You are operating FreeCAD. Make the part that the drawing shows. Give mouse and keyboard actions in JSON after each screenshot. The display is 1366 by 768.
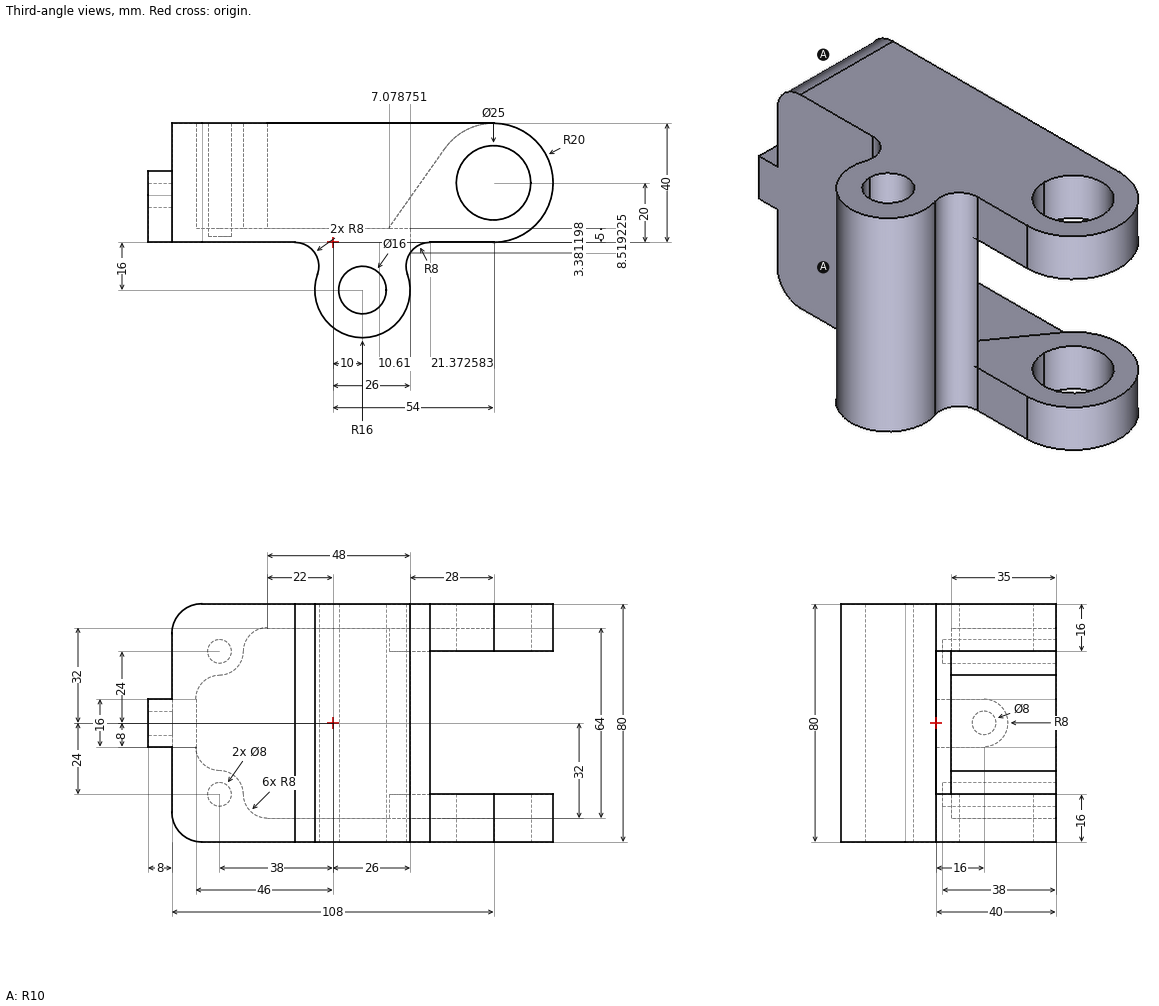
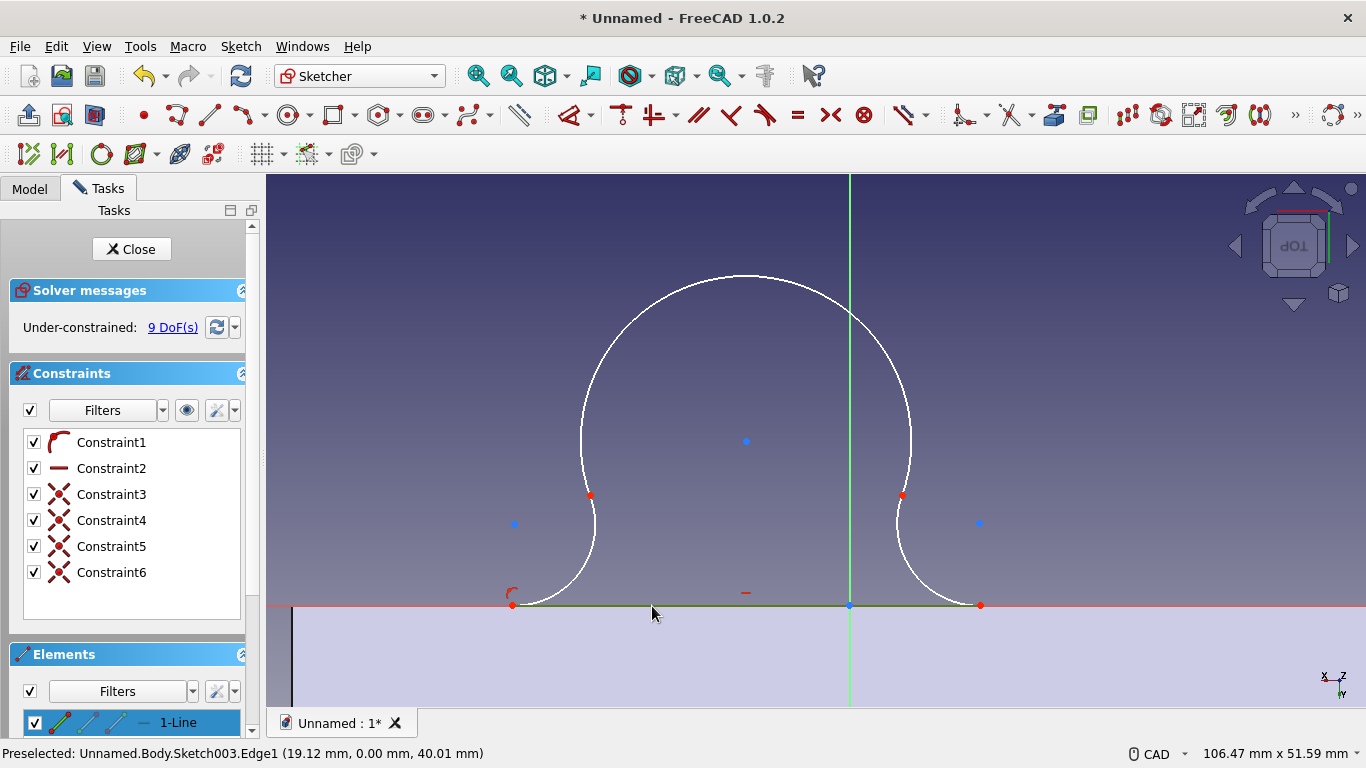
{"action": "left_click", "coordinate": [899, 543]}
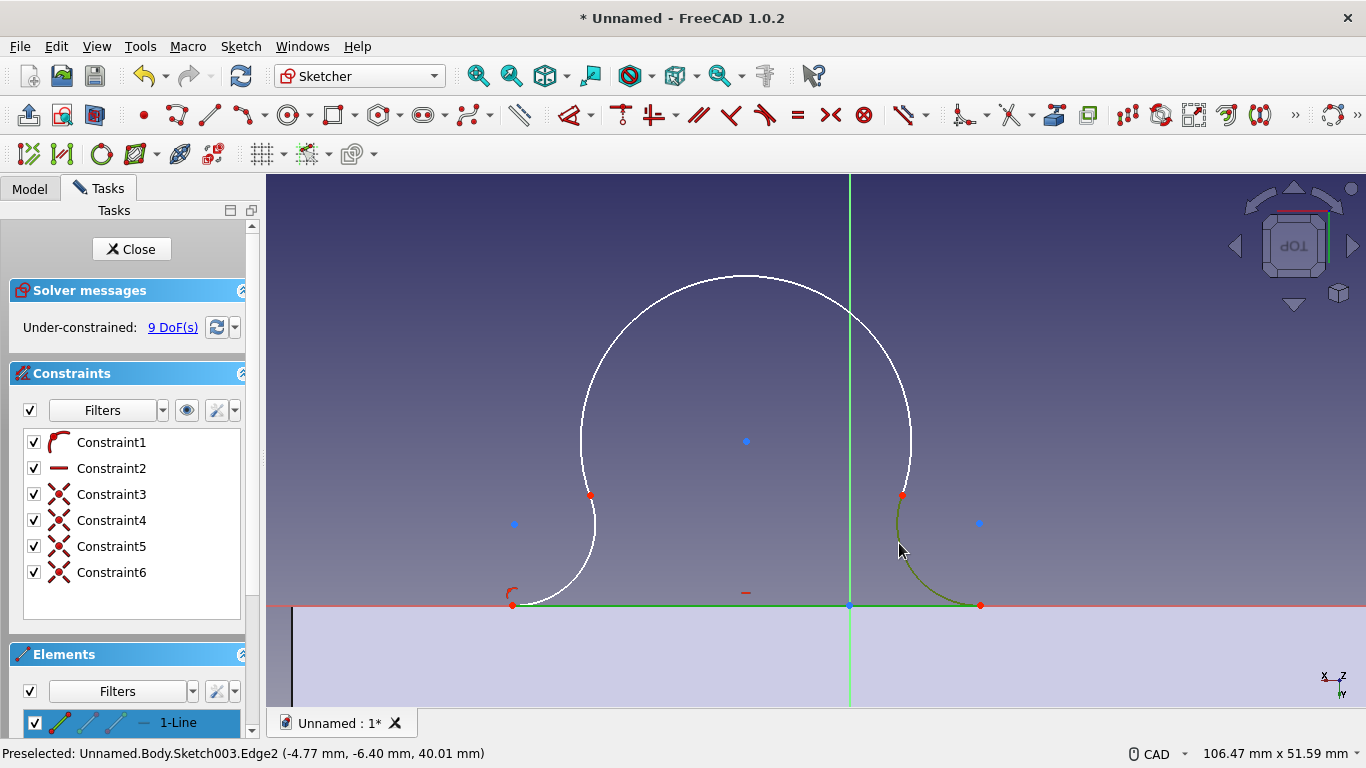
{"action": "key", "text": "t"}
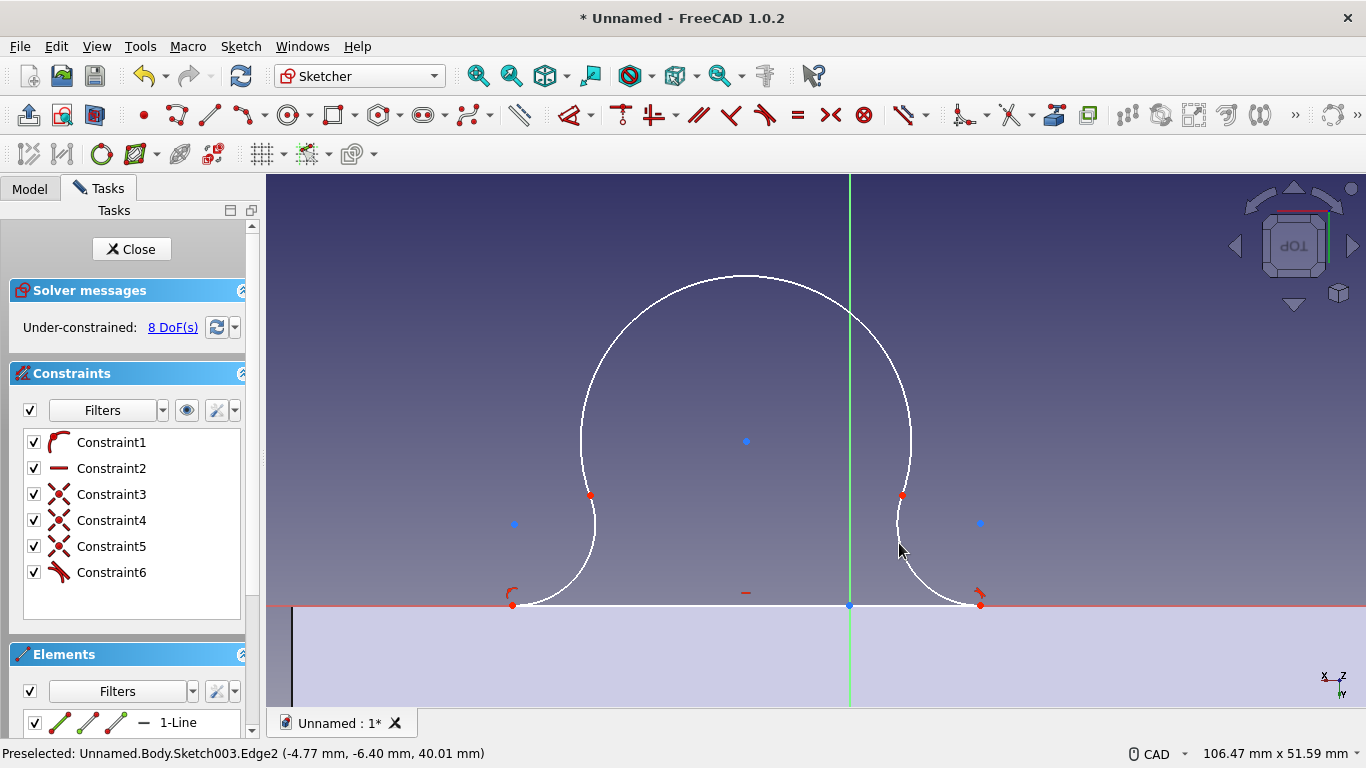
{"action": "left_click", "coordinate": [652, 606]}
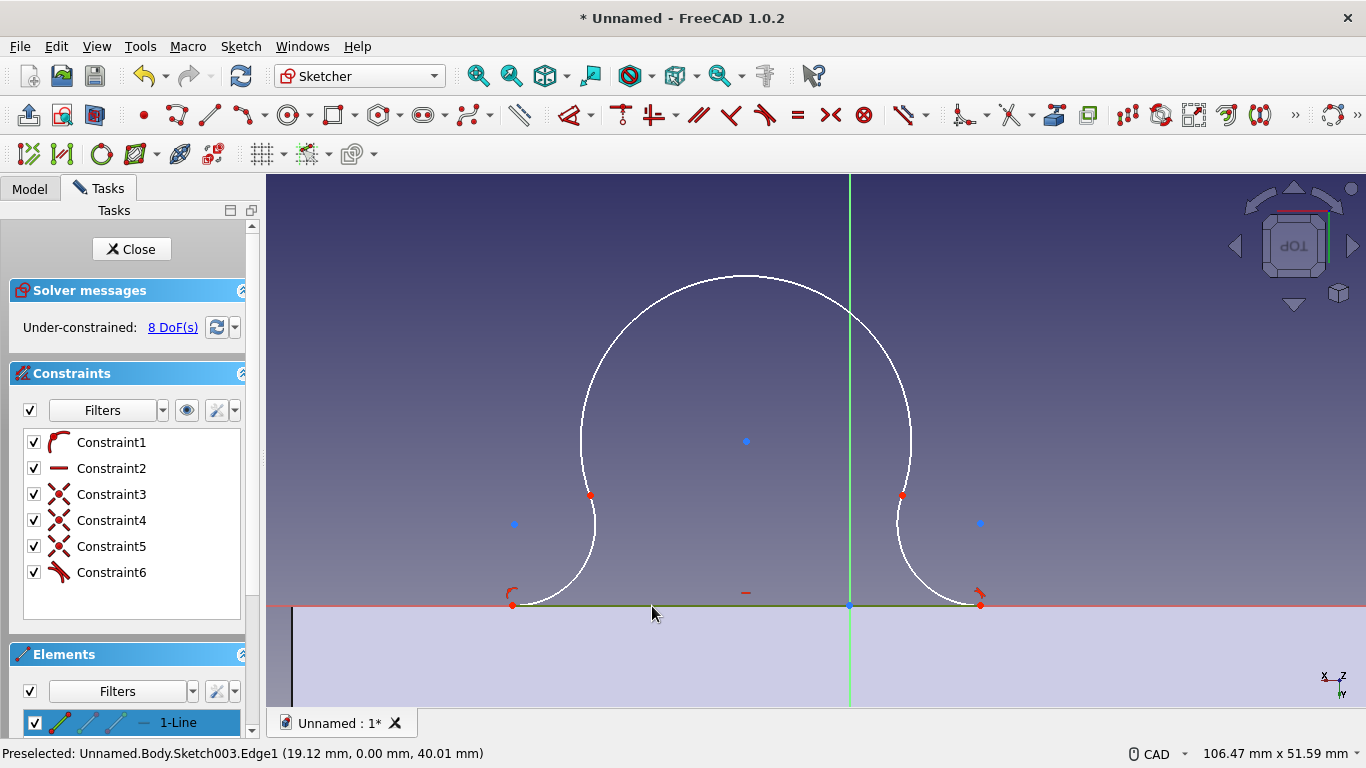
{"action": "left_click", "coordinate": [557, 593]}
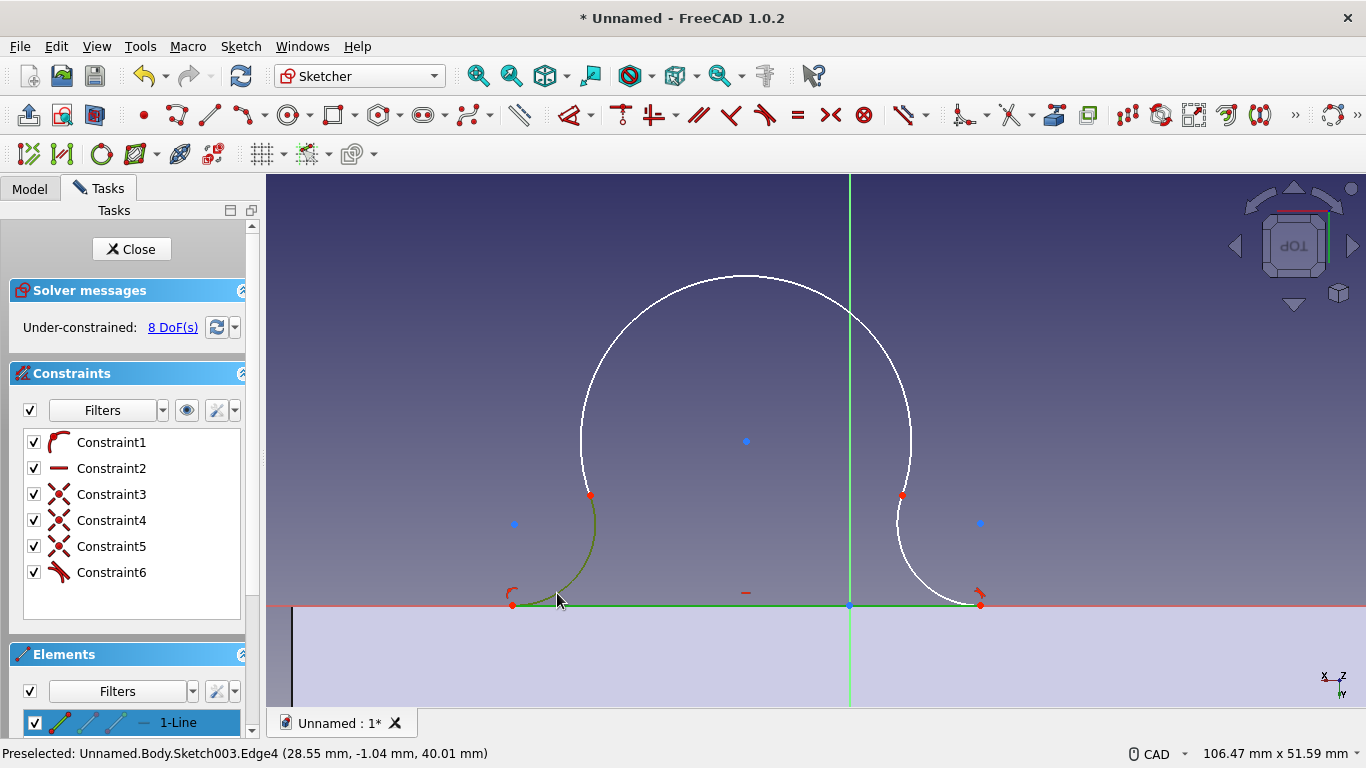
{"action": "left_click", "coordinate": [765, 116]}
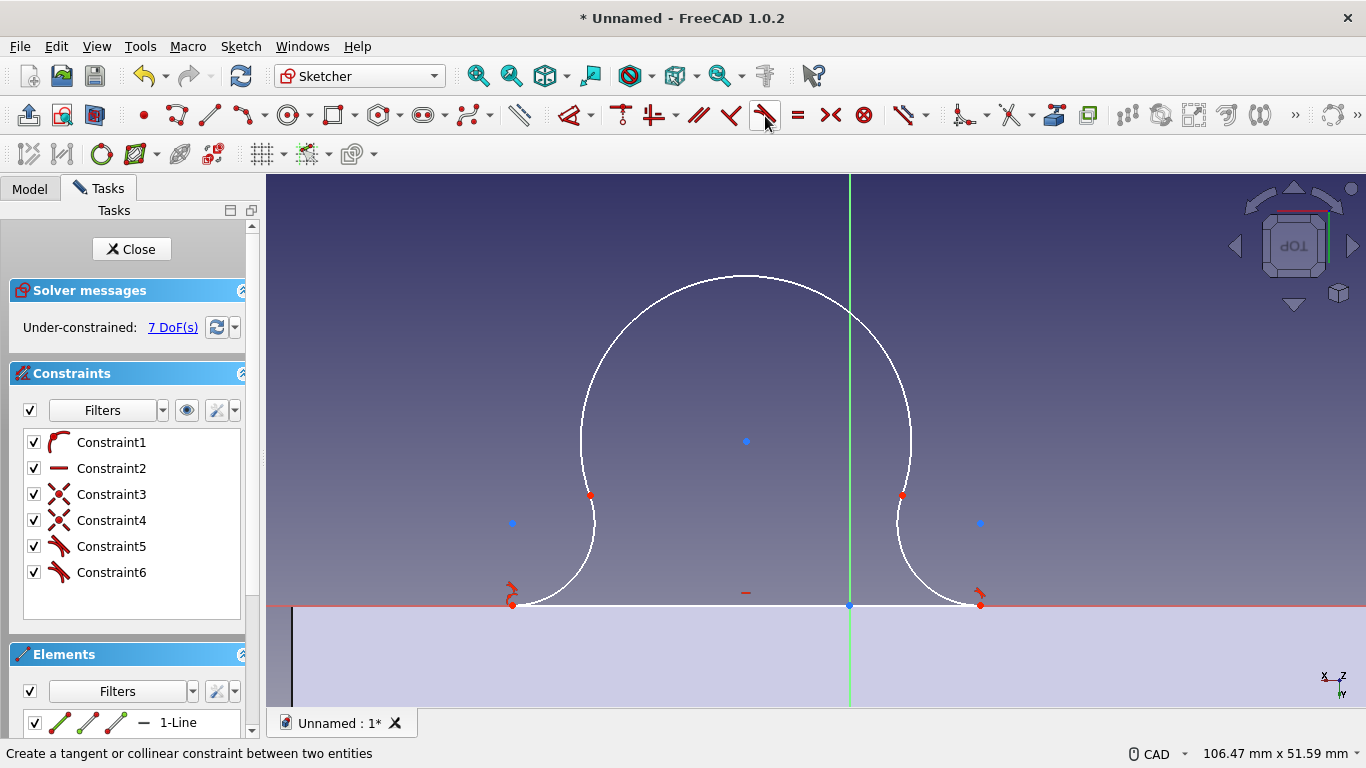
{"action": "left_click", "coordinate": [900, 543]}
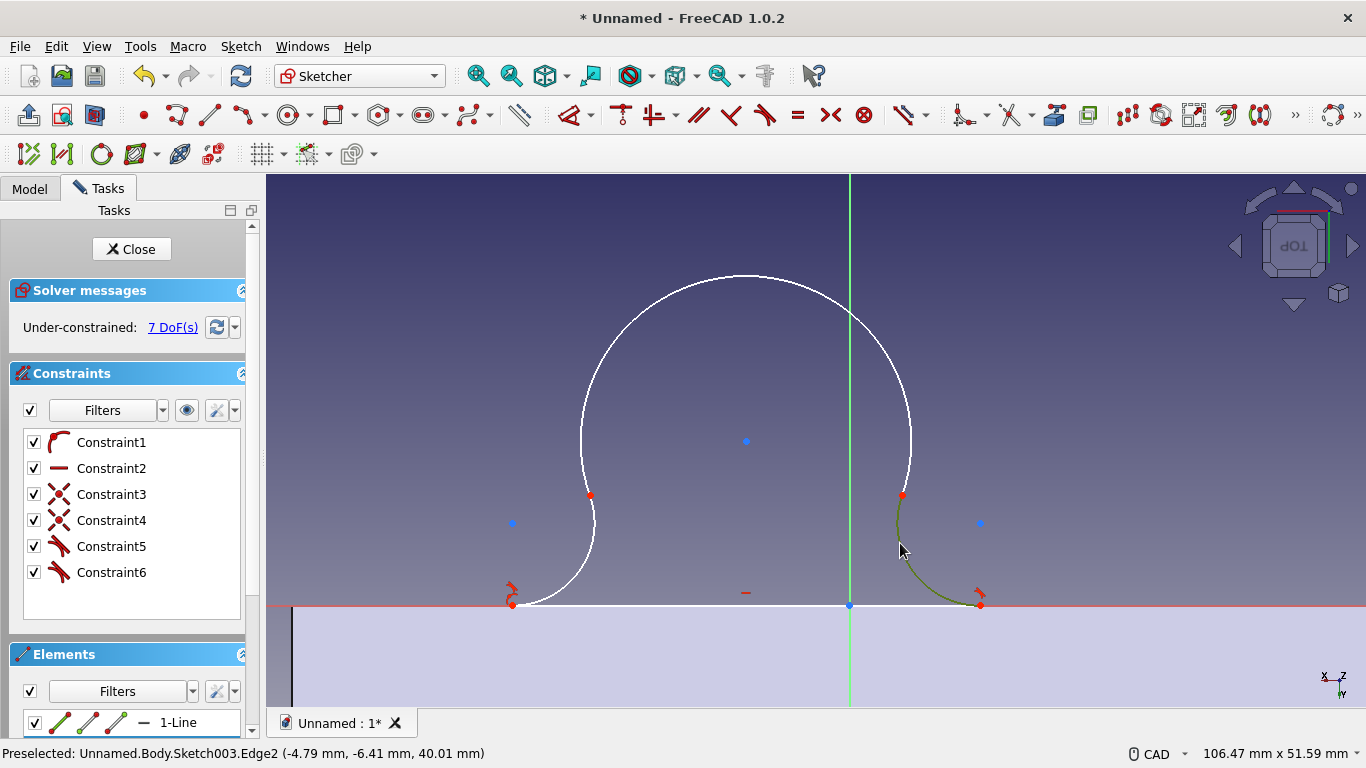
{"action": "scroll", "coordinate": [860, 322], "scroll_direction": "up", "scroll_amount": 2}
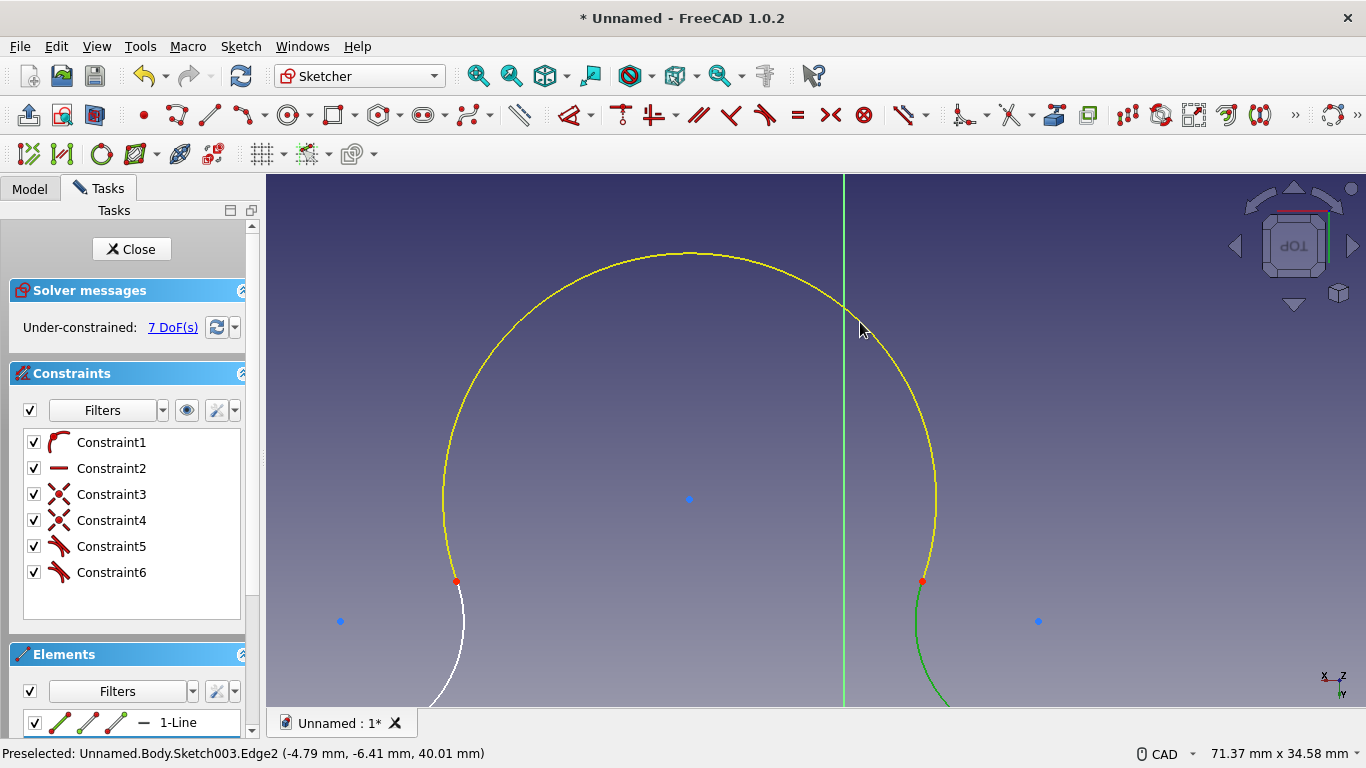
{"action": "left_click", "coordinate": [860, 322]}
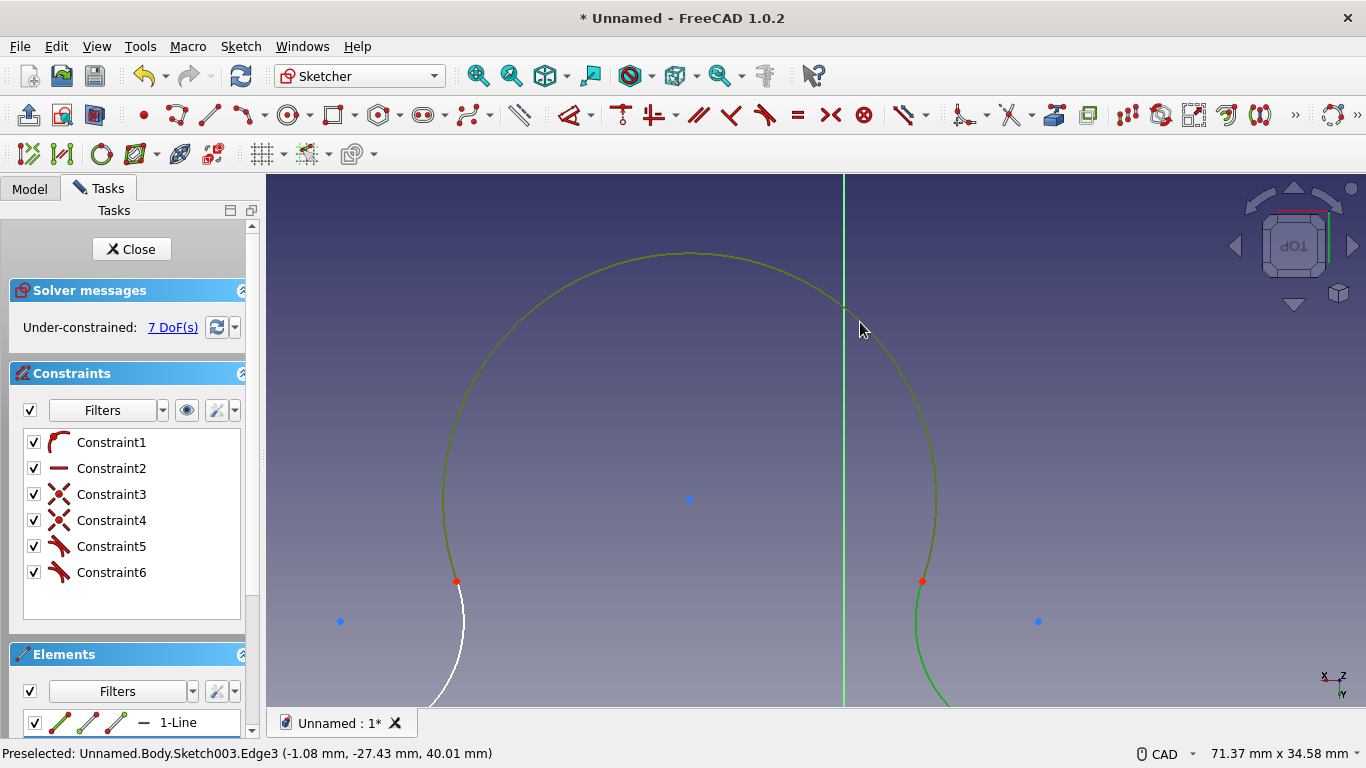
{"action": "left_click", "coordinate": [765, 116]}